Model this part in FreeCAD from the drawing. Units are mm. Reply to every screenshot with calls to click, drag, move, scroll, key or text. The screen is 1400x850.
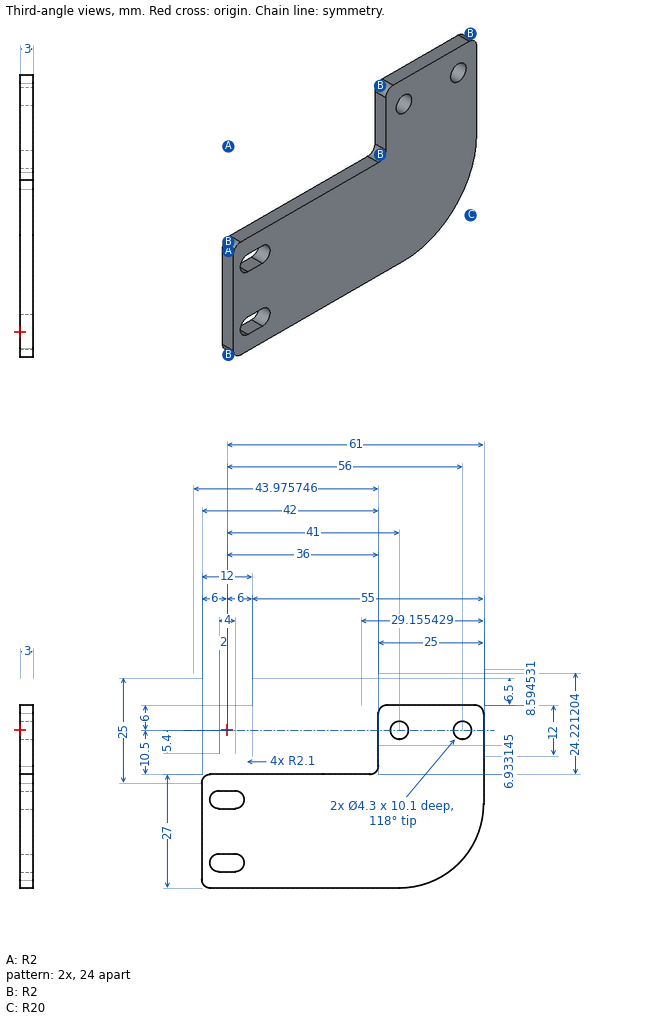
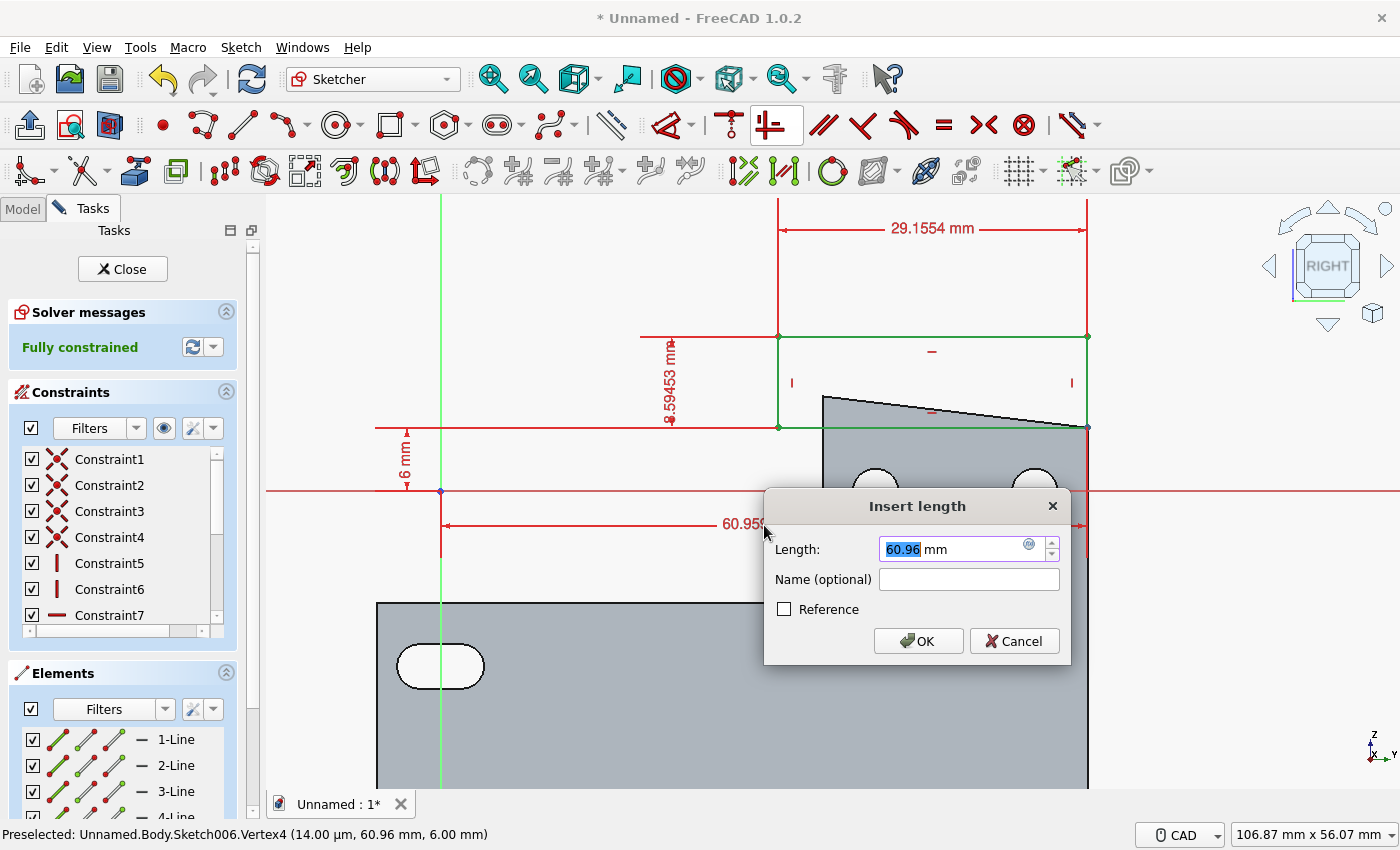
text(61)
key(Return)
key(Escape)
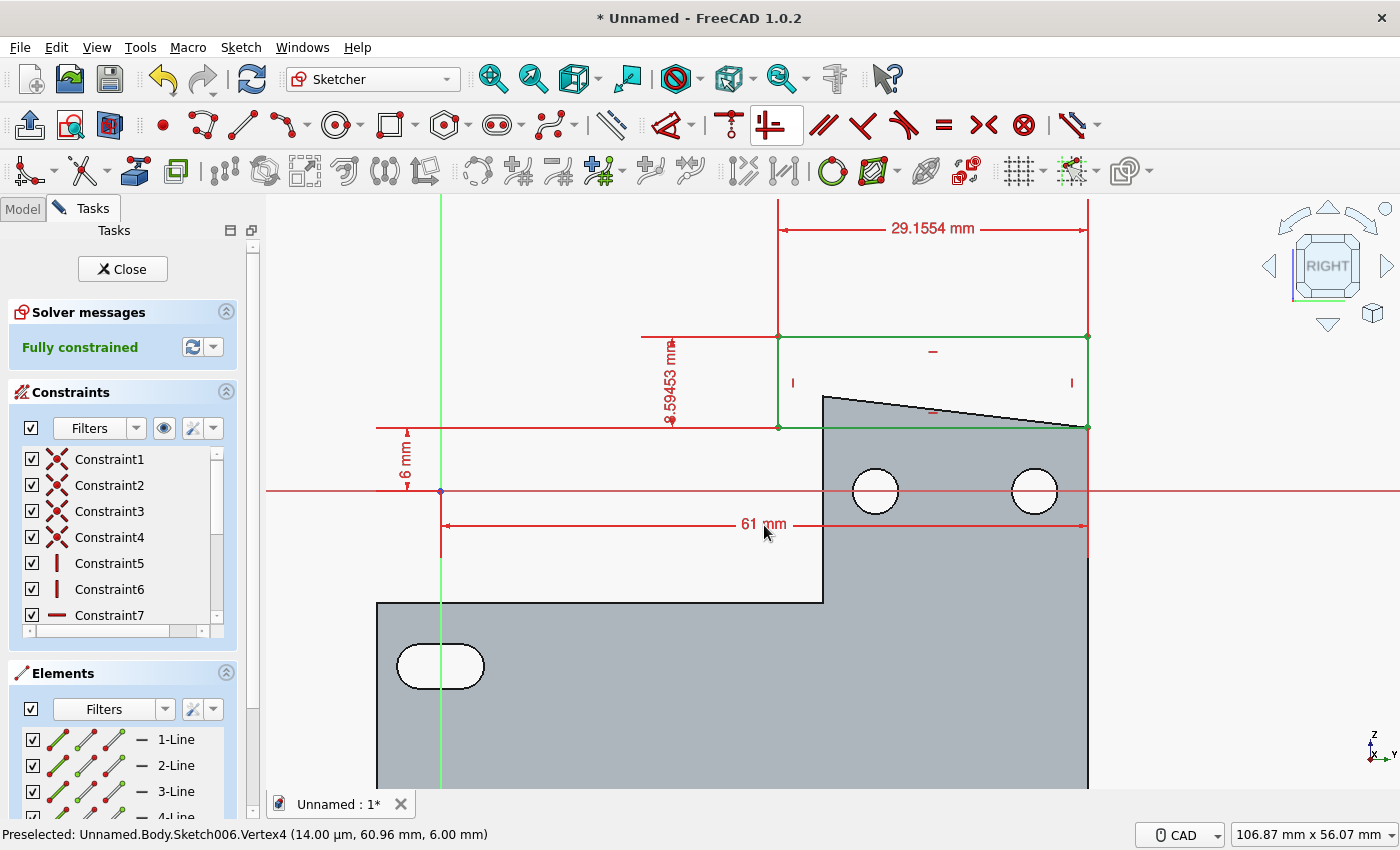
click(123, 269)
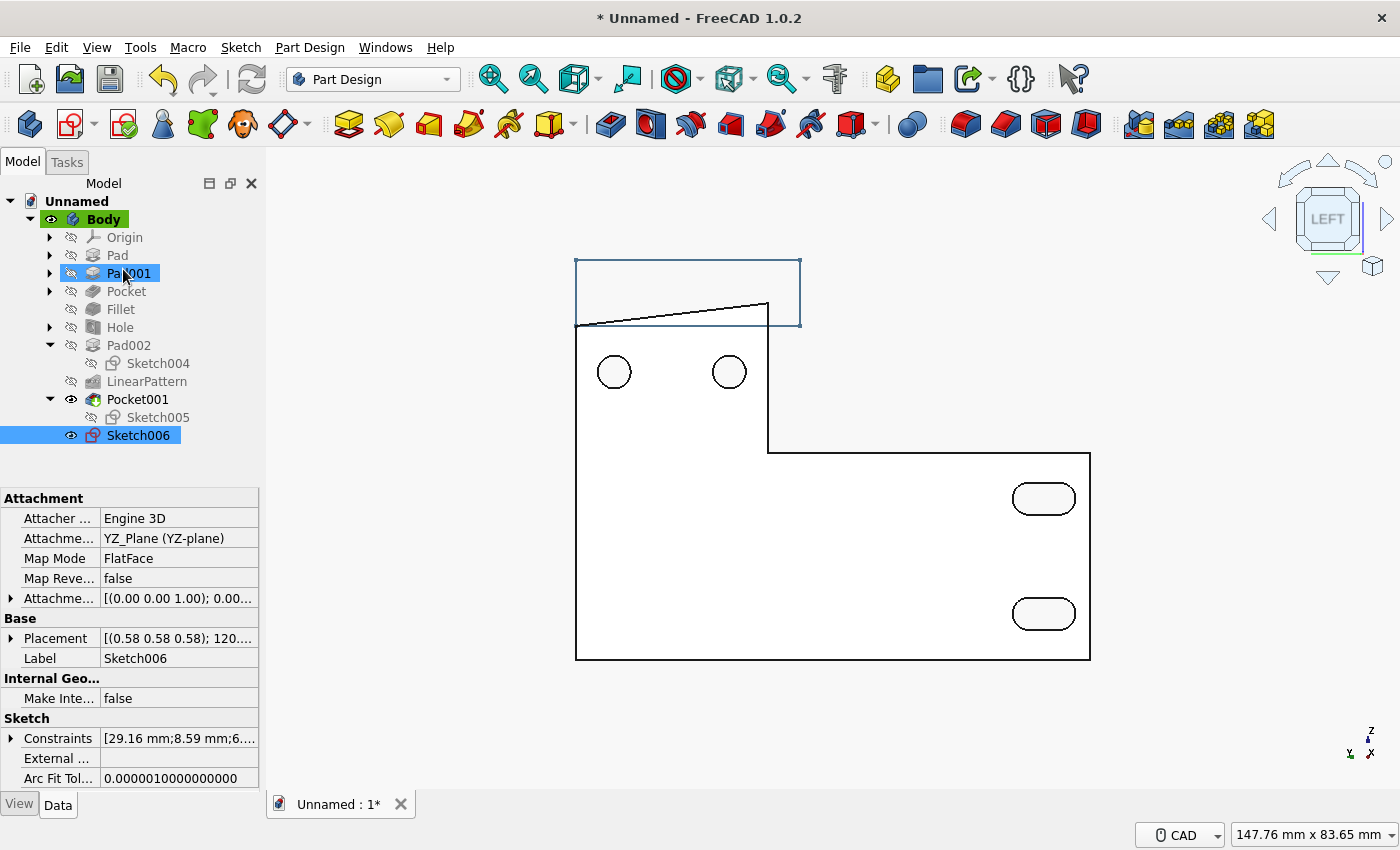
click(612, 124)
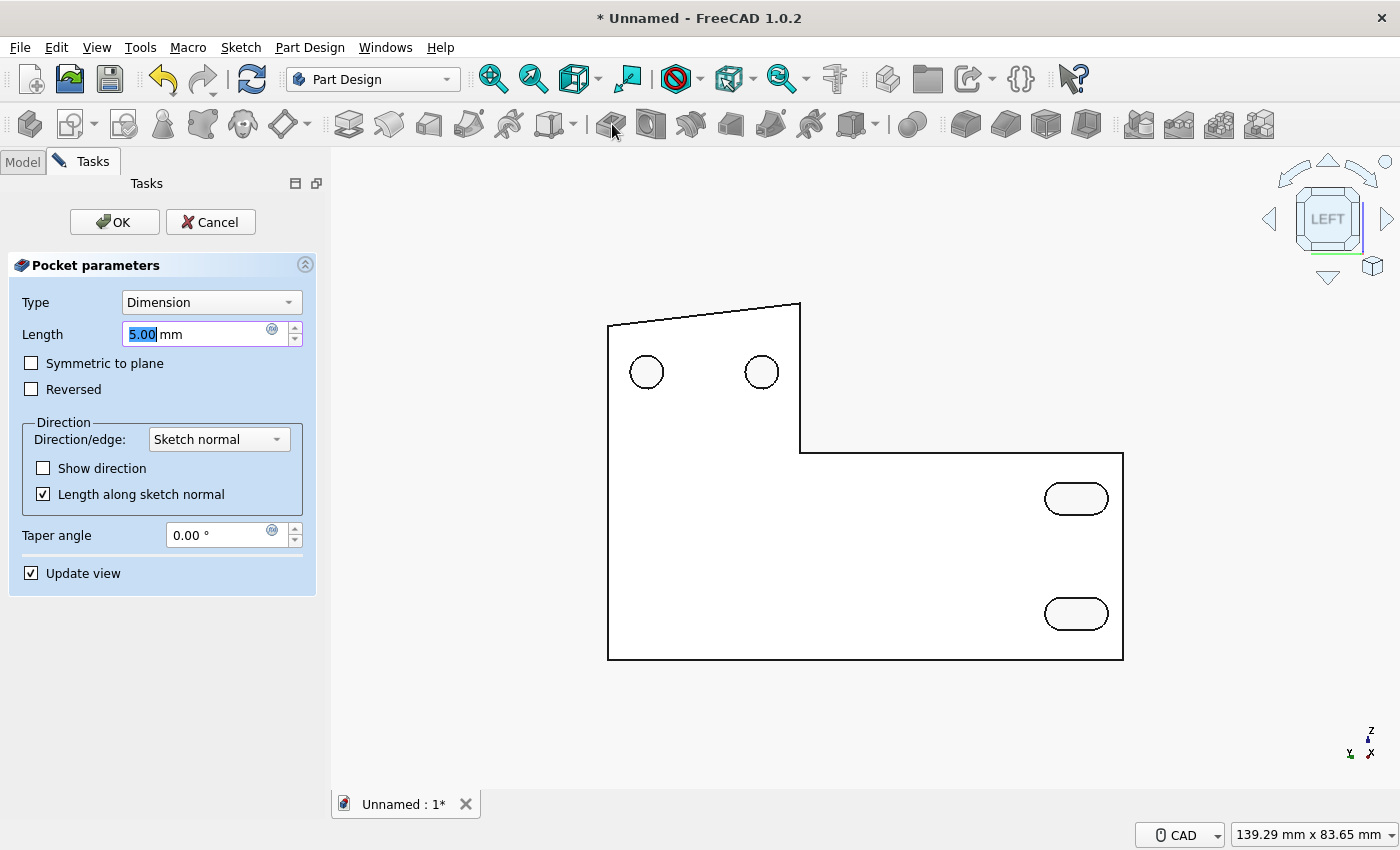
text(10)
key(Tab)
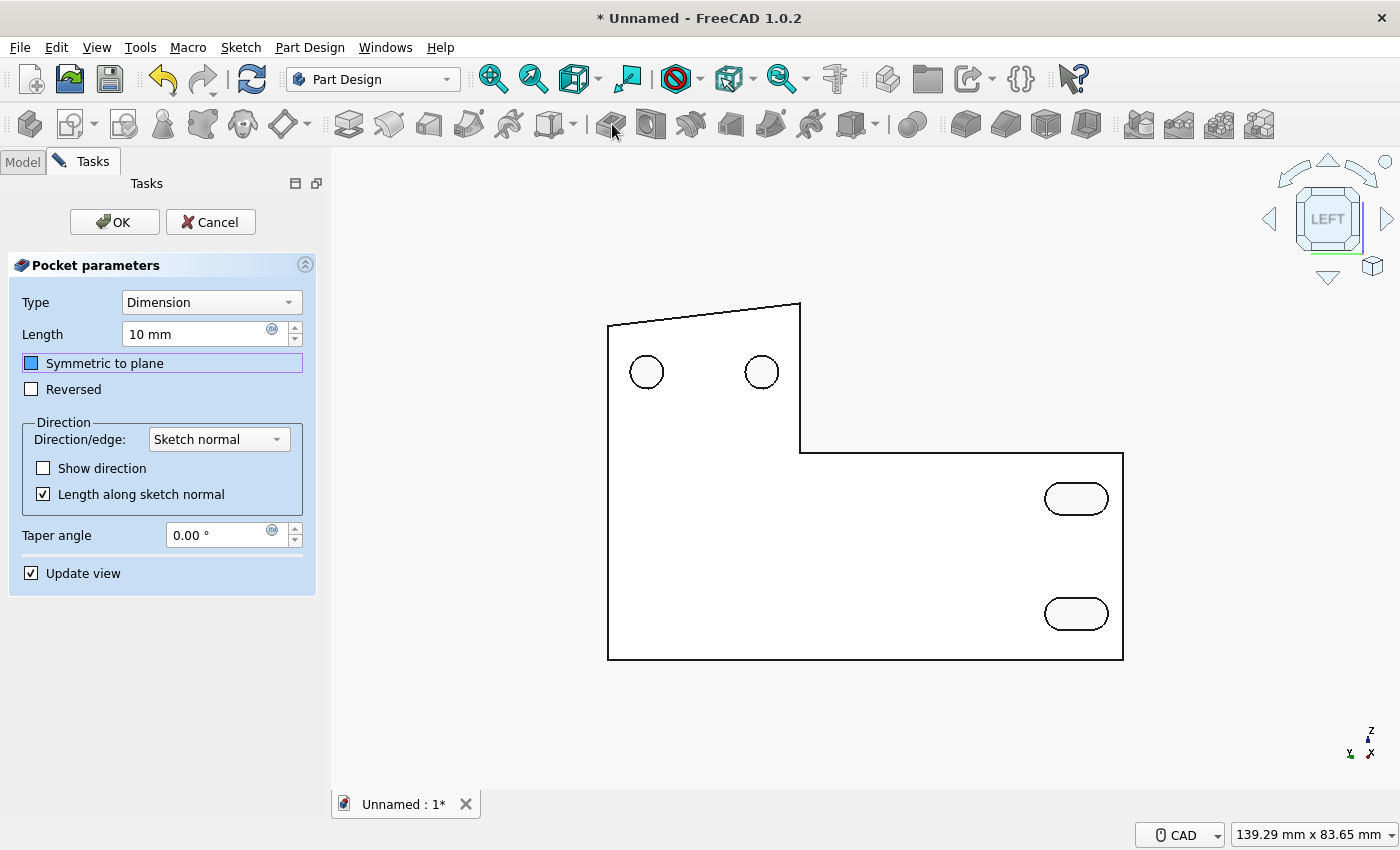
click(30, 389)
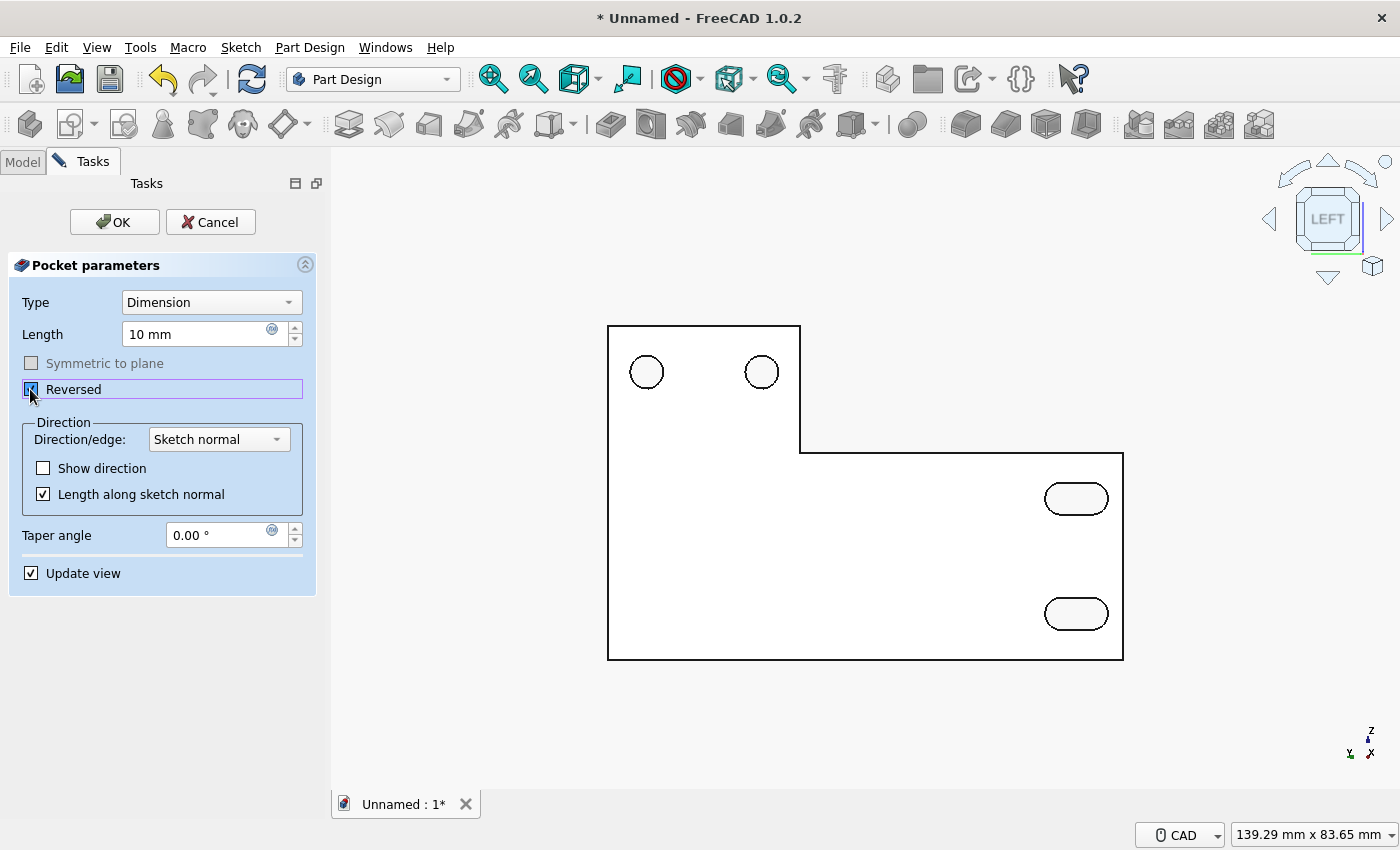
click(115, 222)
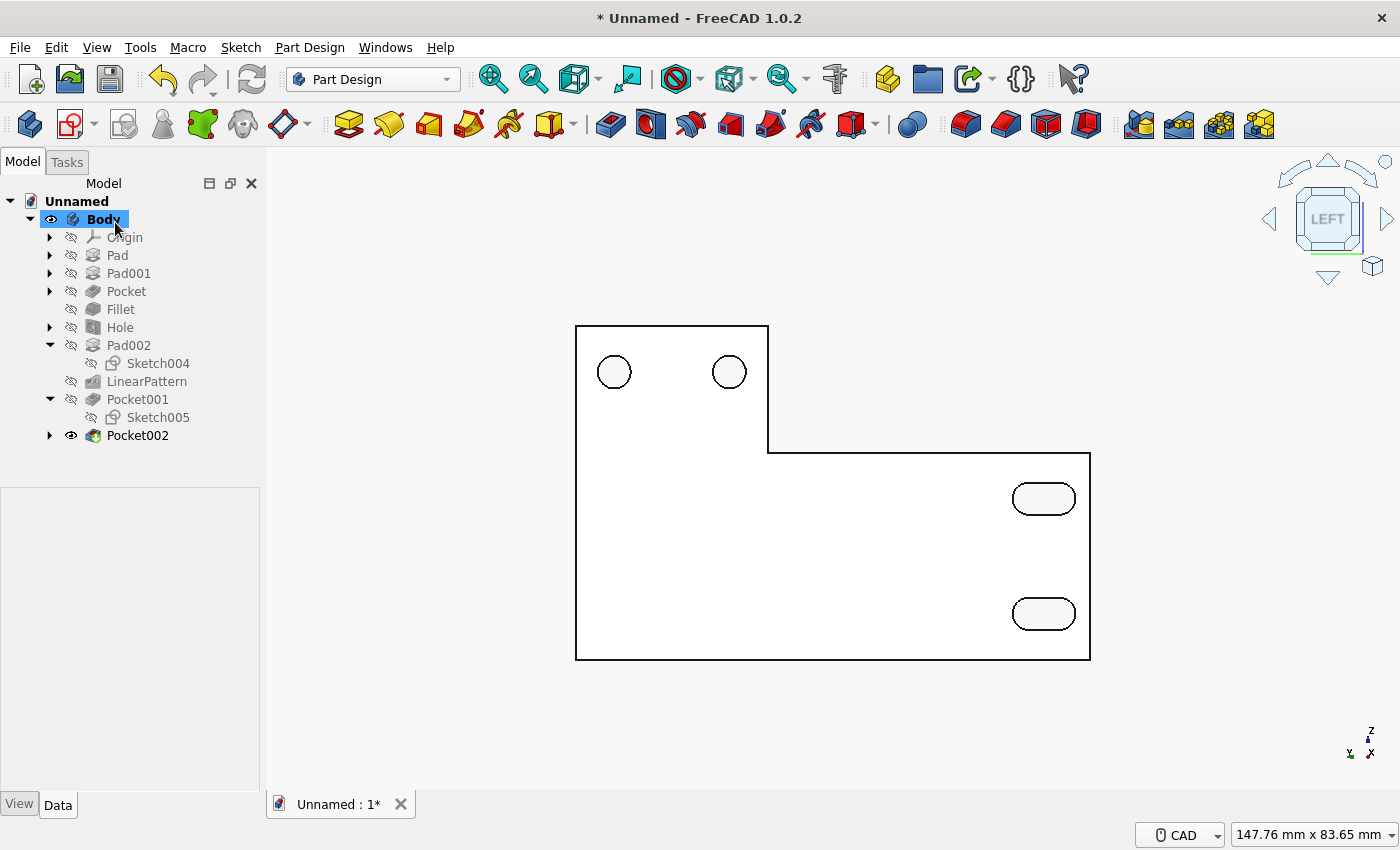
key(0)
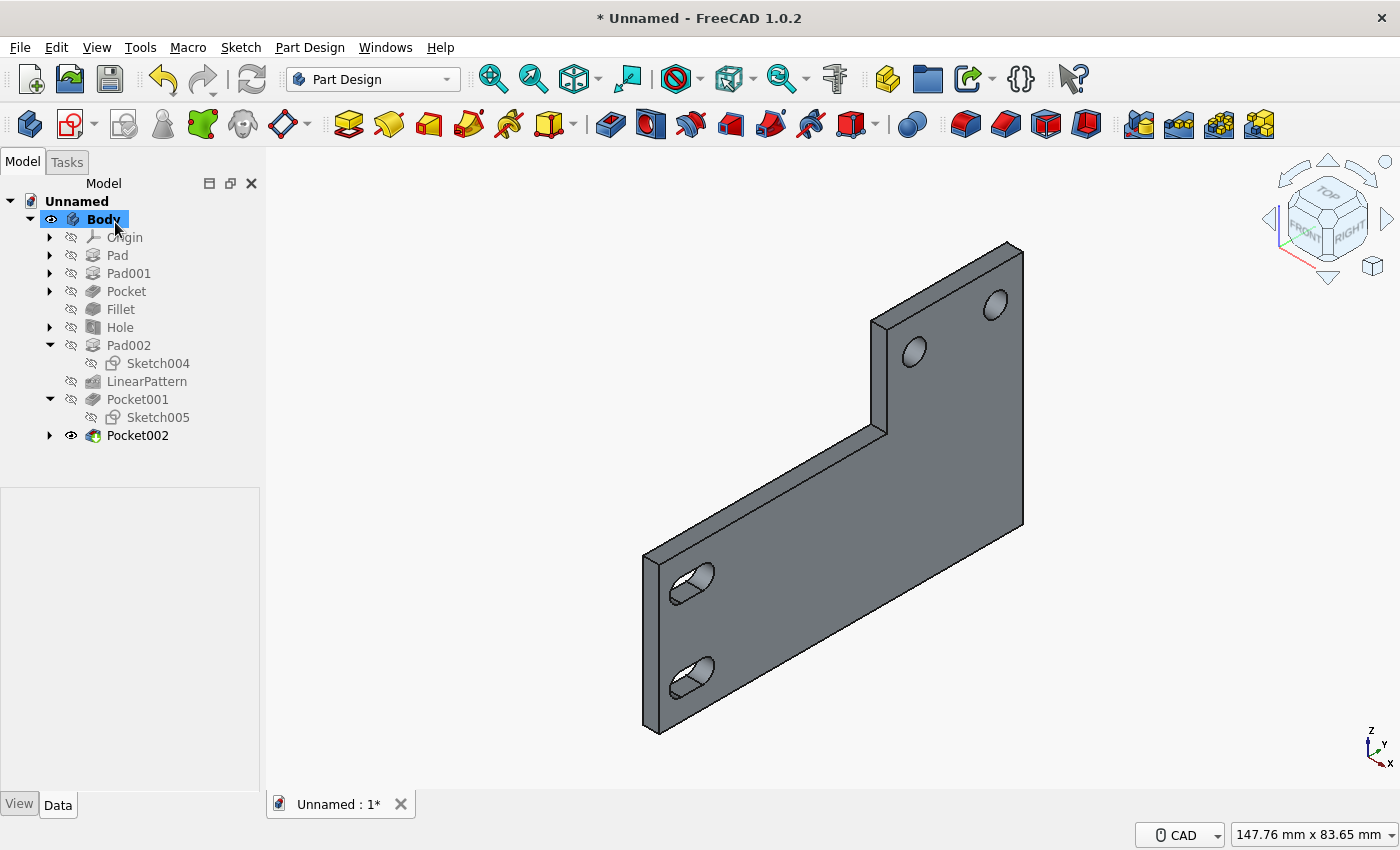
click(651, 559)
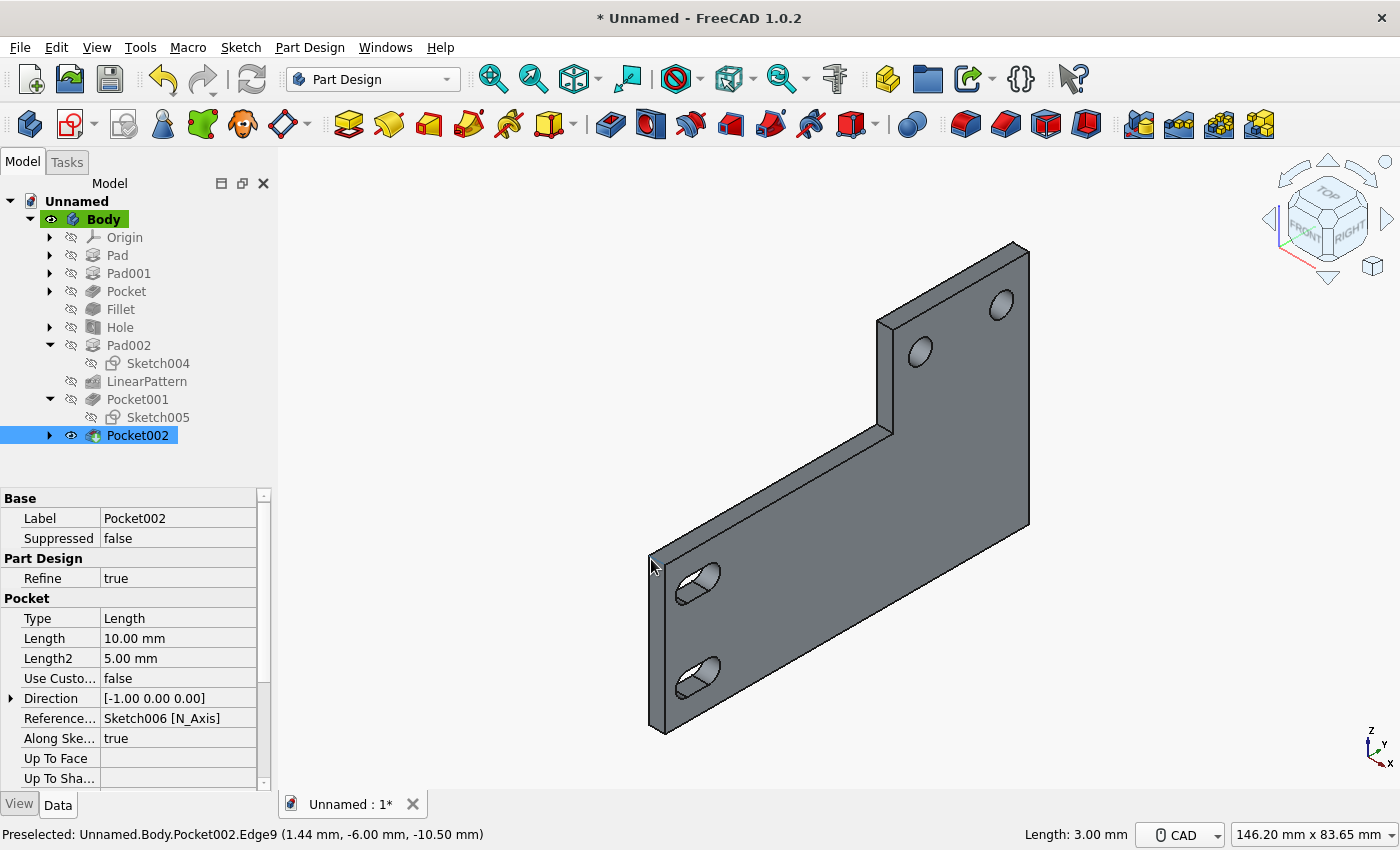
click(885, 324, ctrl)